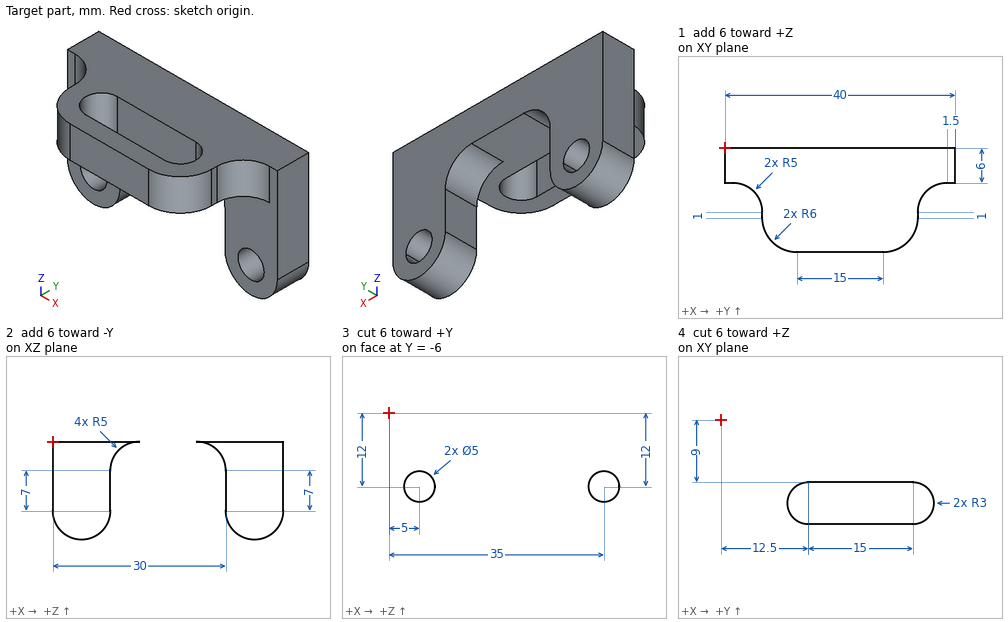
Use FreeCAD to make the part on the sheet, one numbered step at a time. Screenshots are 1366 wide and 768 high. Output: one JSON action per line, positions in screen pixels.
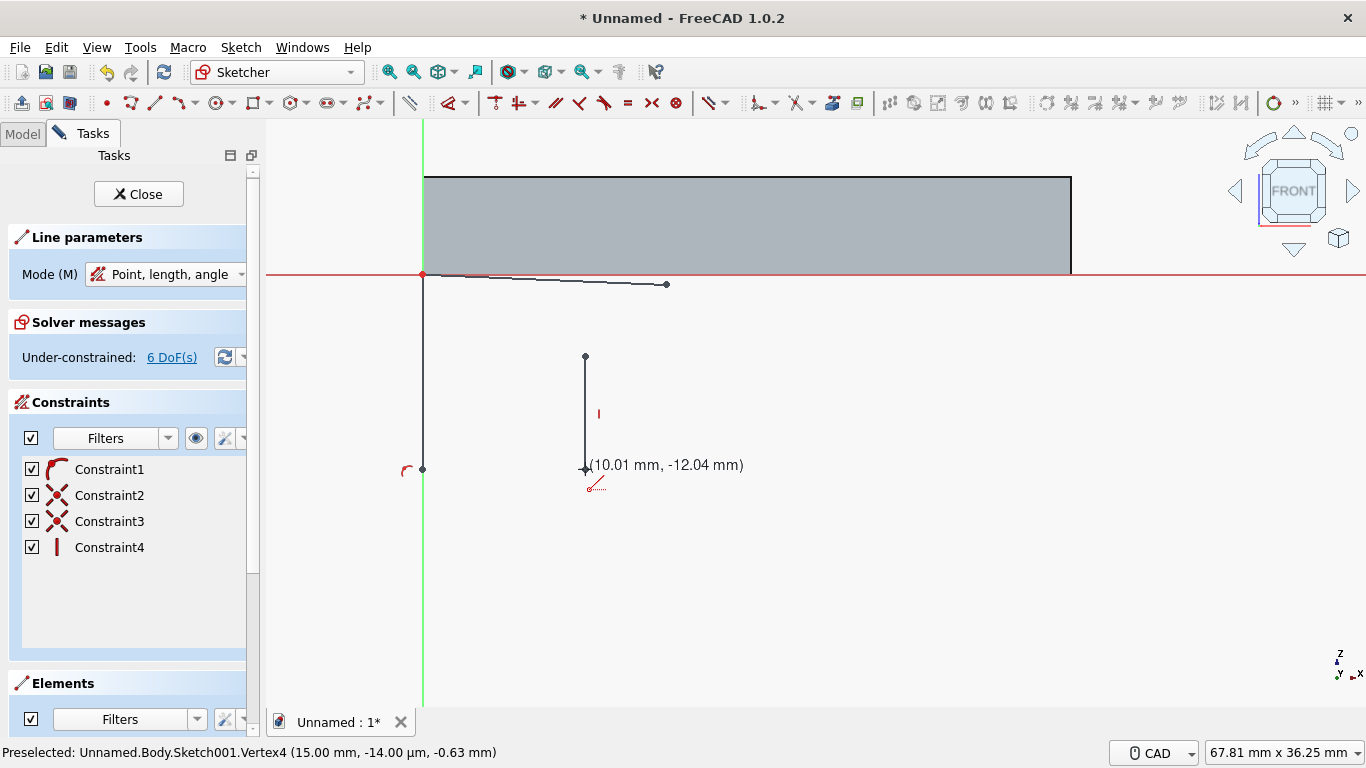
{"action": "key", "text": "g 3 a"}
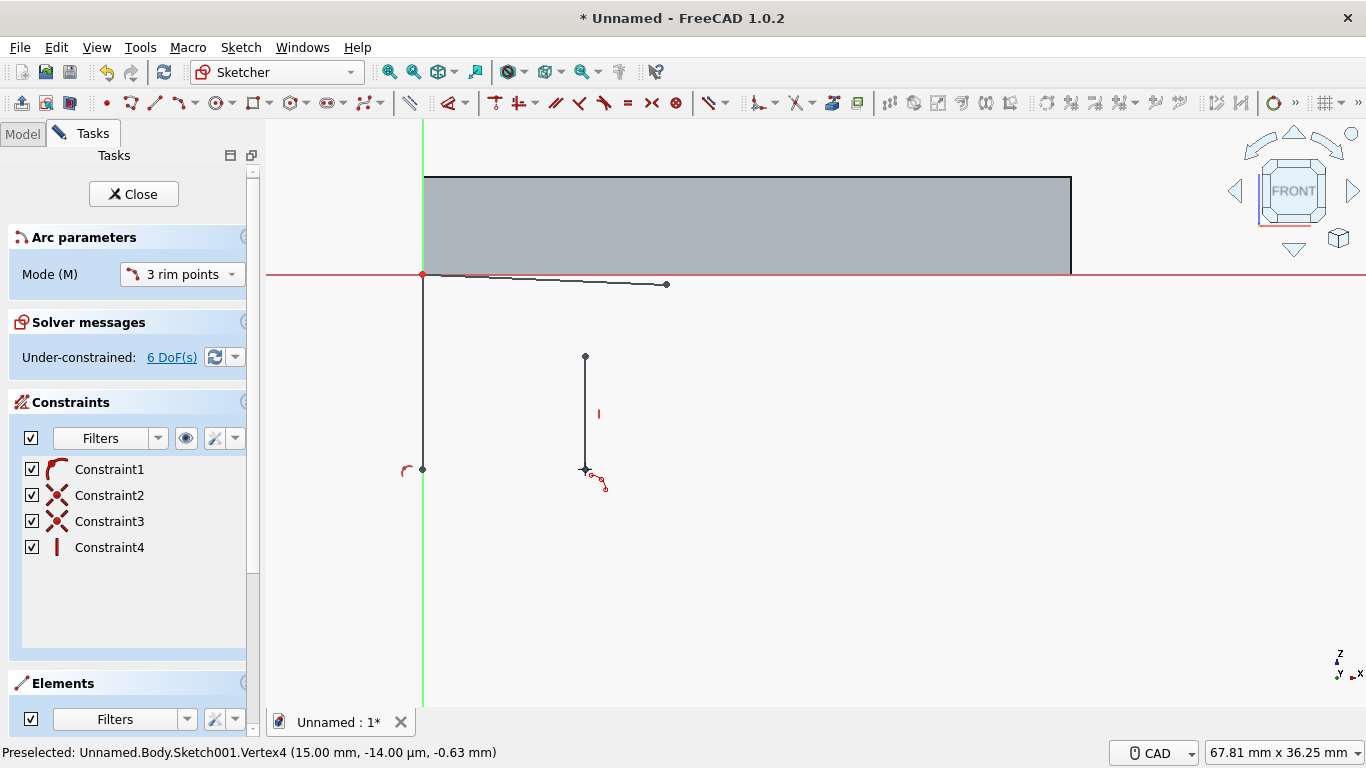
{"action": "left_click", "coordinate": [666, 285]}
{"action": "left_click", "coordinate": [585, 357]}
{"action": "left_click", "coordinate": [609, 298]}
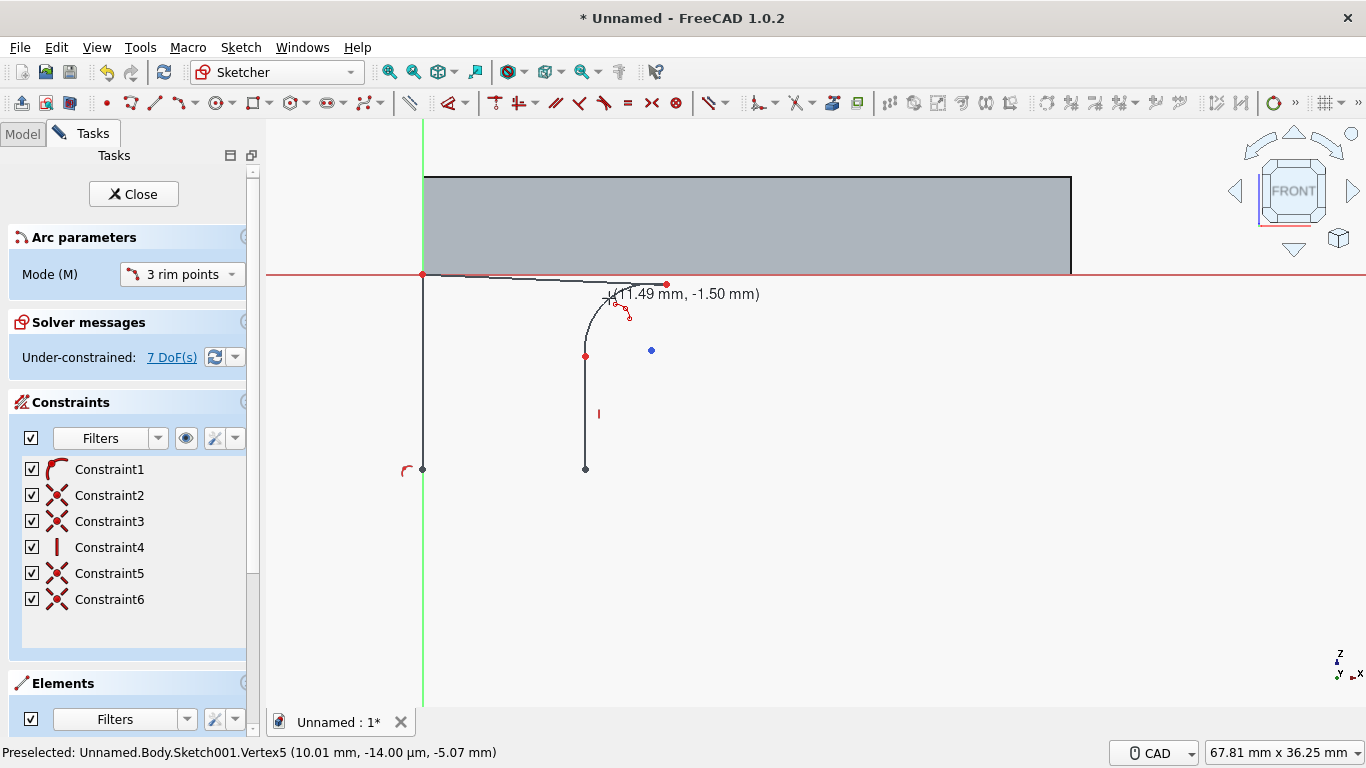
{"action": "left_click", "coordinate": [585, 470]}
{"action": "left_click", "coordinate": [423, 470]}
{"action": "left_click", "coordinate": [504, 550]}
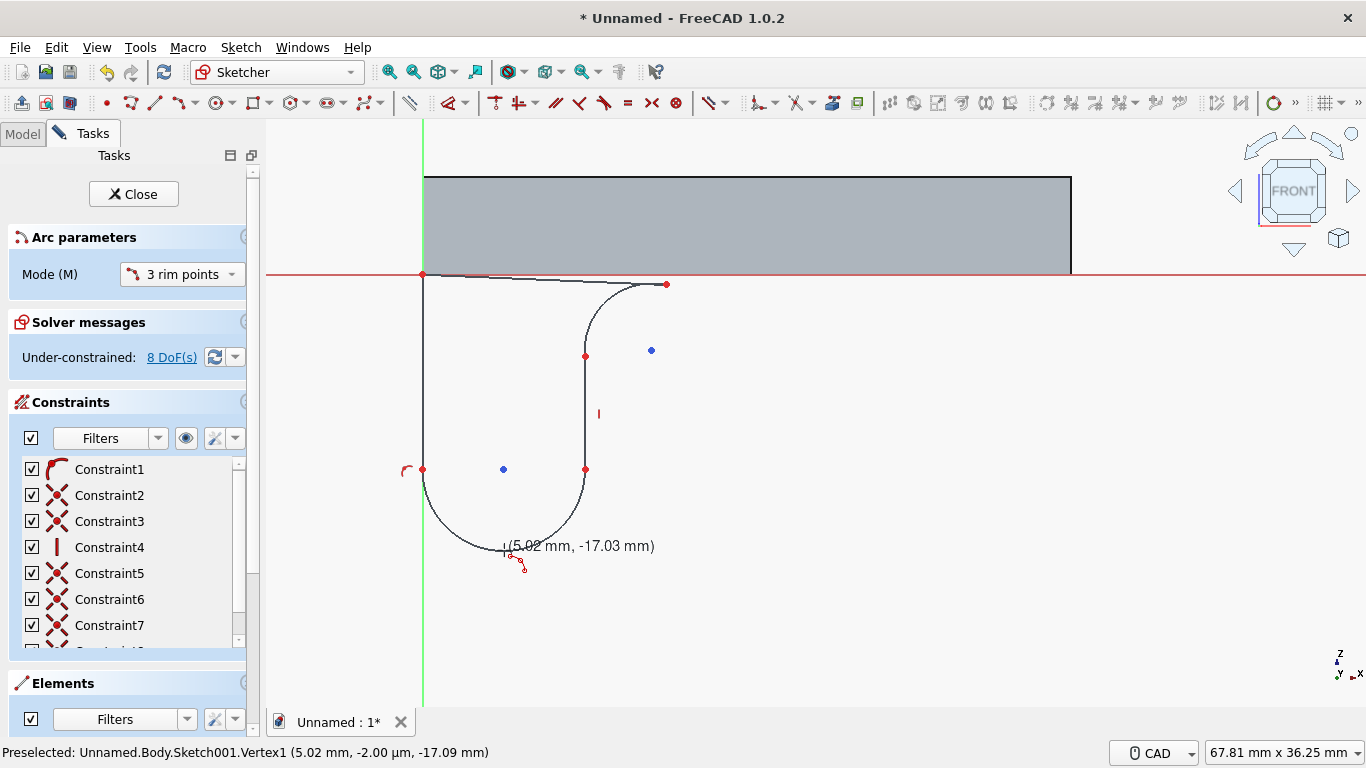
{"action": "left_click", "coordinate": [156, 104]}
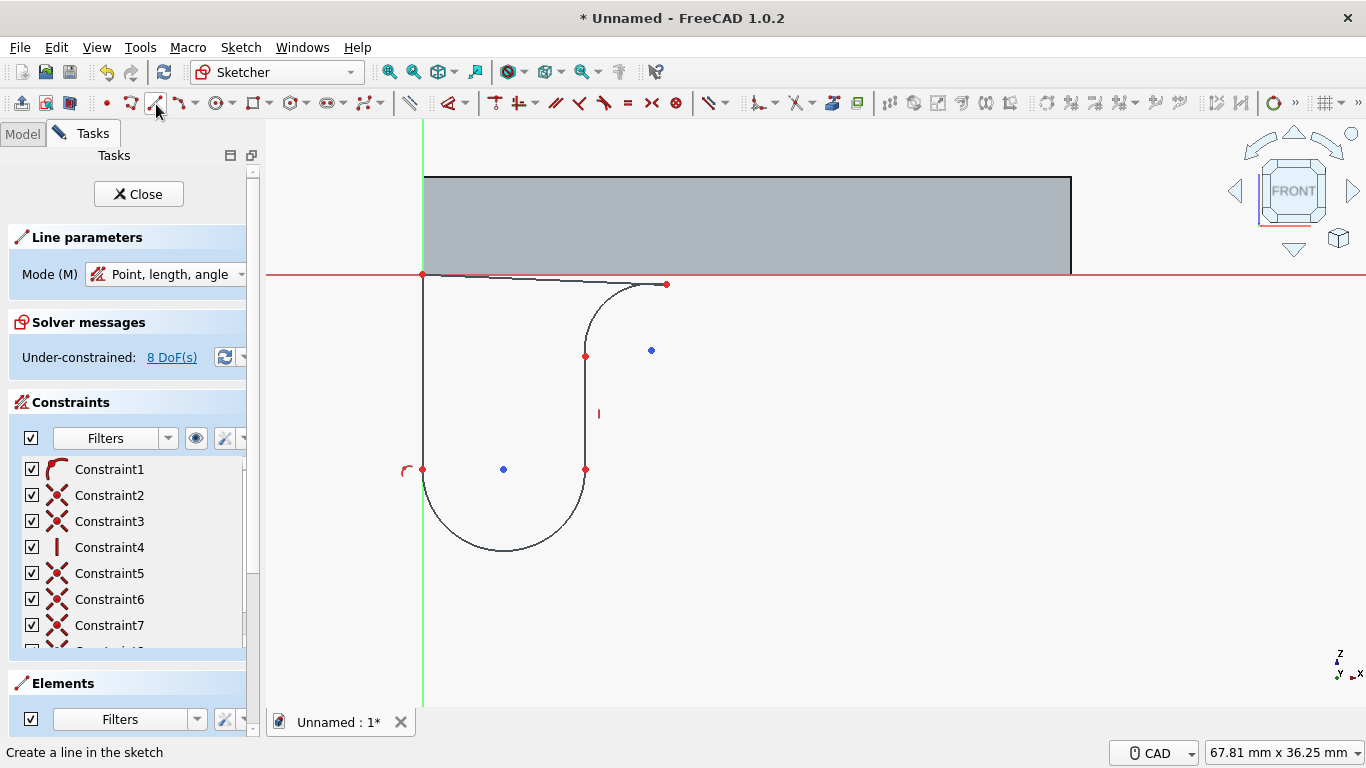
{"action": "left_click", "coordinate": [909, 469]}
{"action": "left_click", "coordinate": [909, 356]}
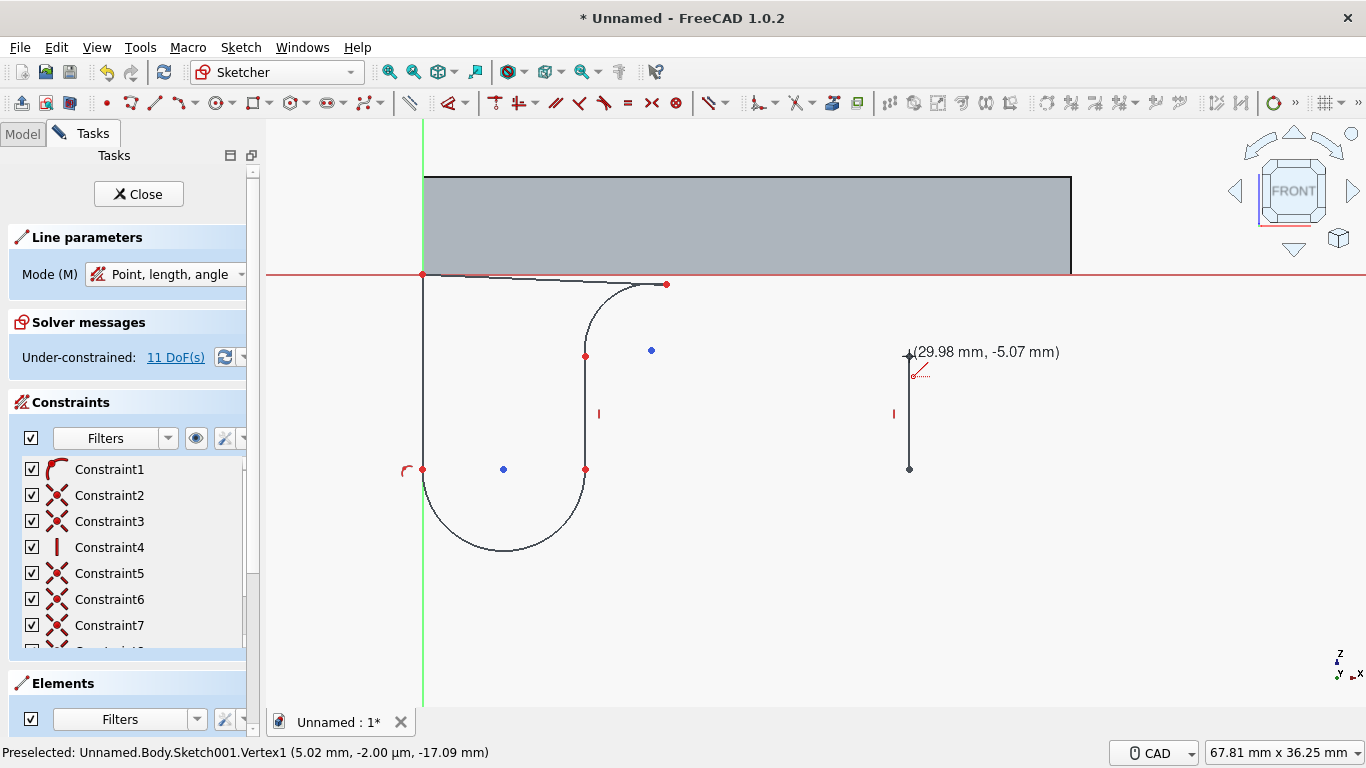
{"action": "key", "text": "g m"}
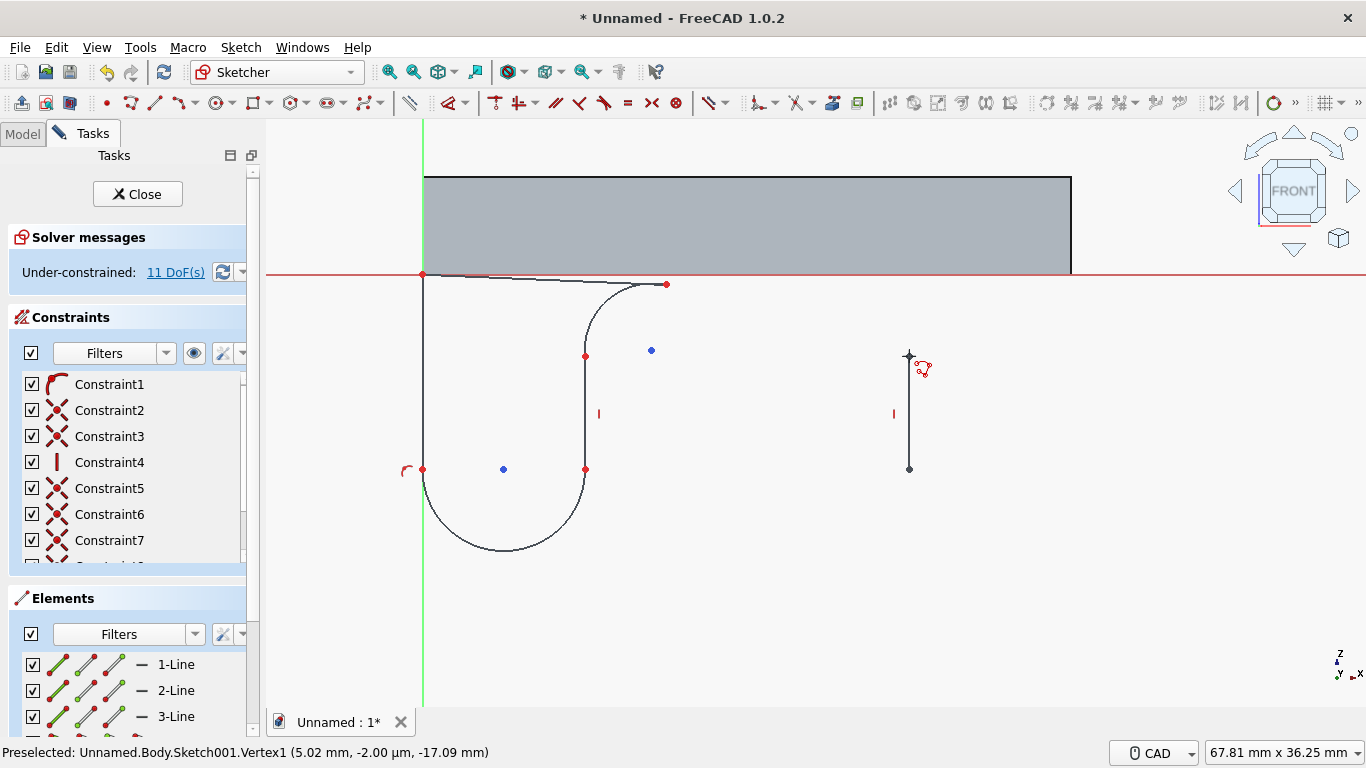
{"action": "left_click", "coordinate": [828, 275]}
{"action": "left_click", "coordinate": [1071, 284]}
{"action": "left_click", "coordinate": [1071, 469]}
{"action": "right_click", "coordinate": [1071, 469]}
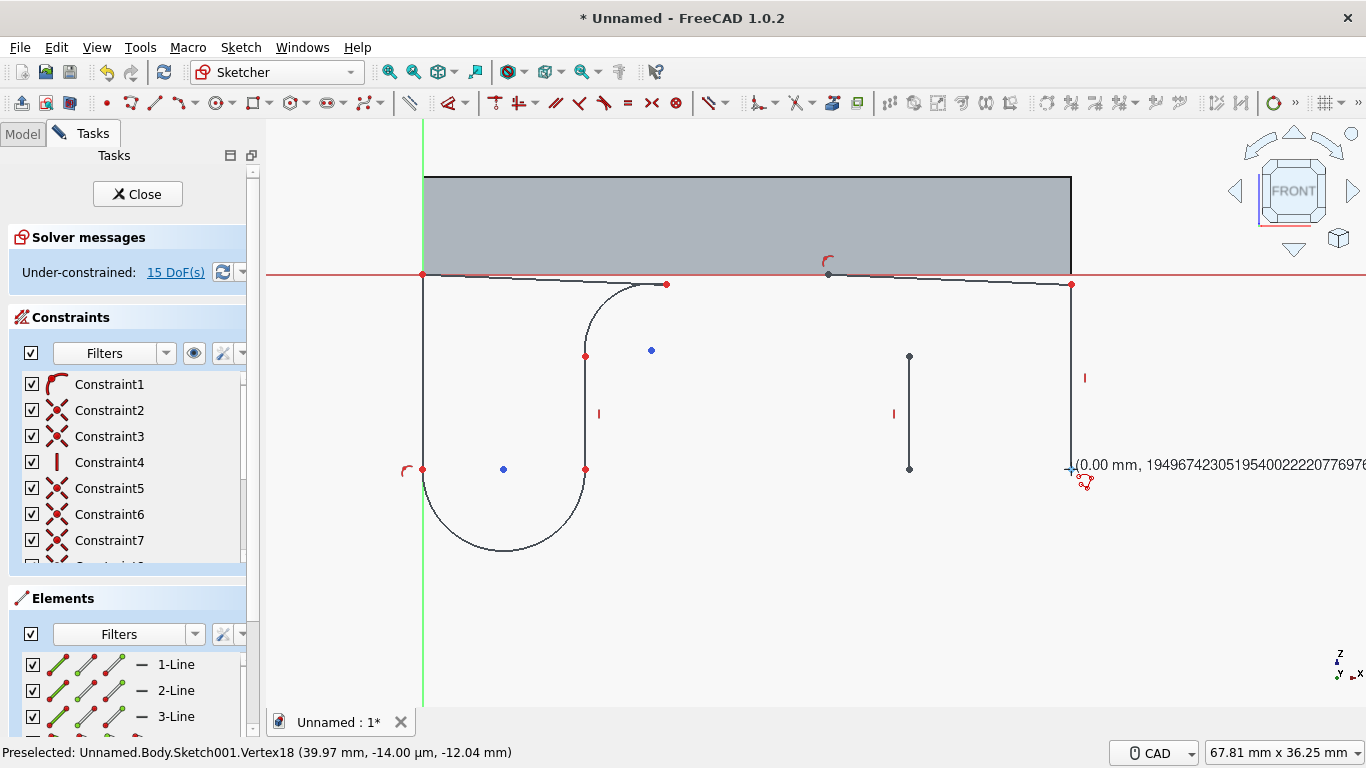
{"action": "left_click", "coordinate": [180, 104]}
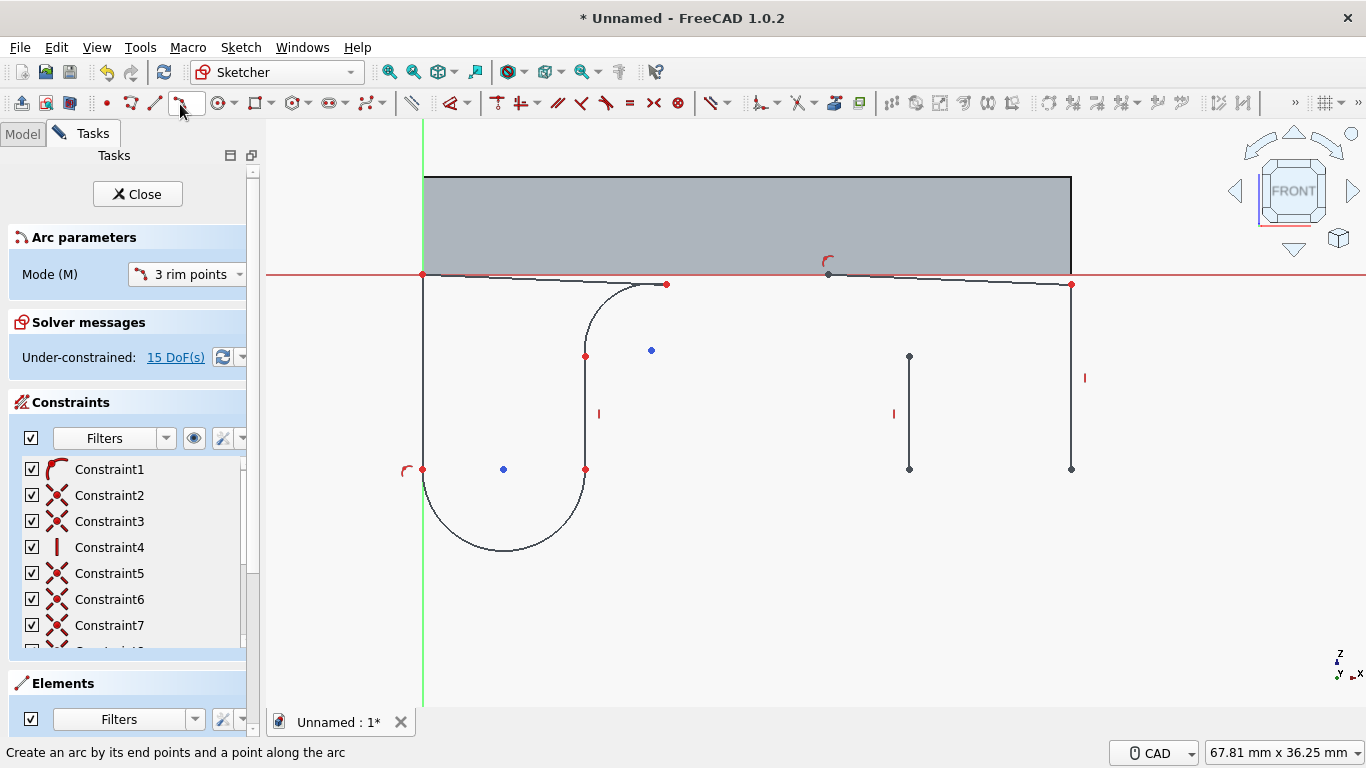
{"action": "left_click", "coordinate": [909, 357]}
{"action": "left_click", "coordinate": [828, 275]}
{"action": "left_click", "coordinate": [886, 298]}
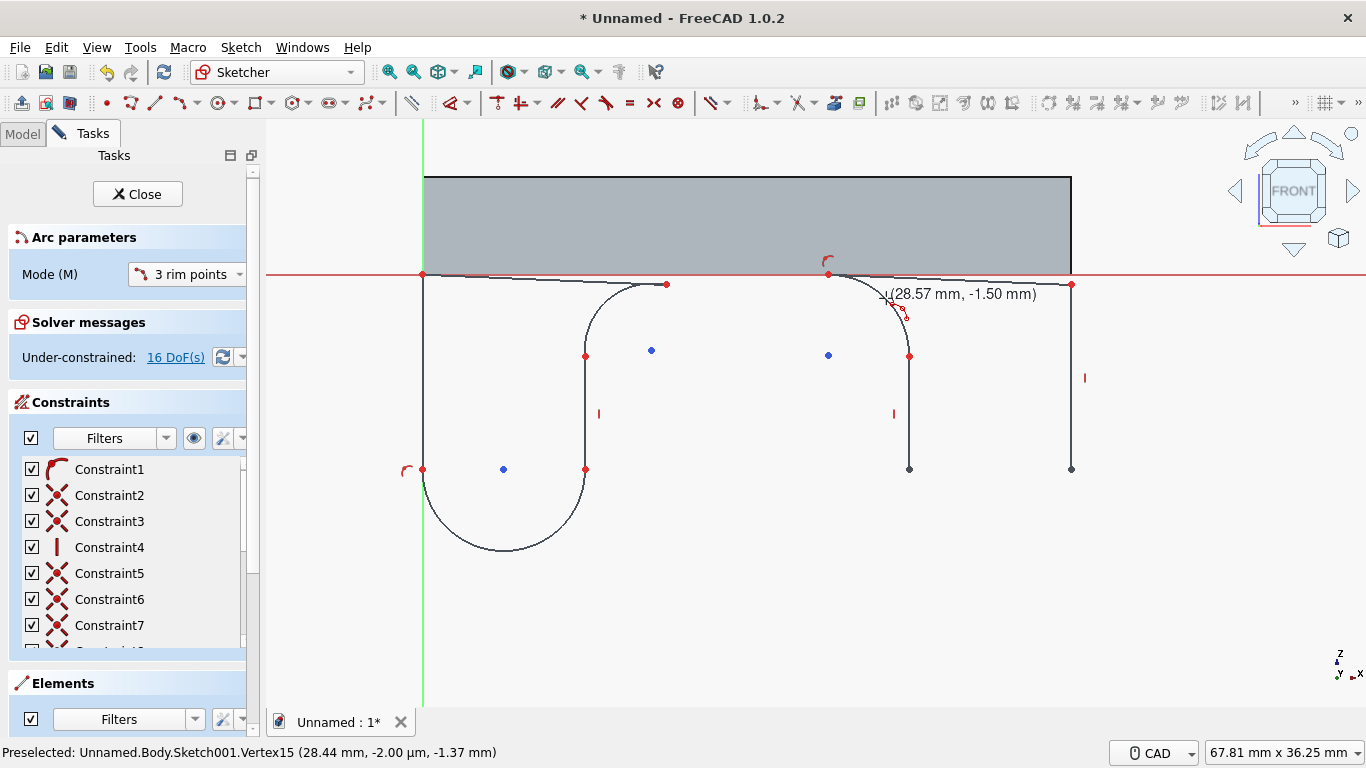
{"action": "left_click", "coordinate": [1071, 470]}
{"action": "left_click", "coordinate": [909, 470]}
{"action": "left_click", "coordinate": [990, 550]}
{"action": "key", "text": "Escape"}